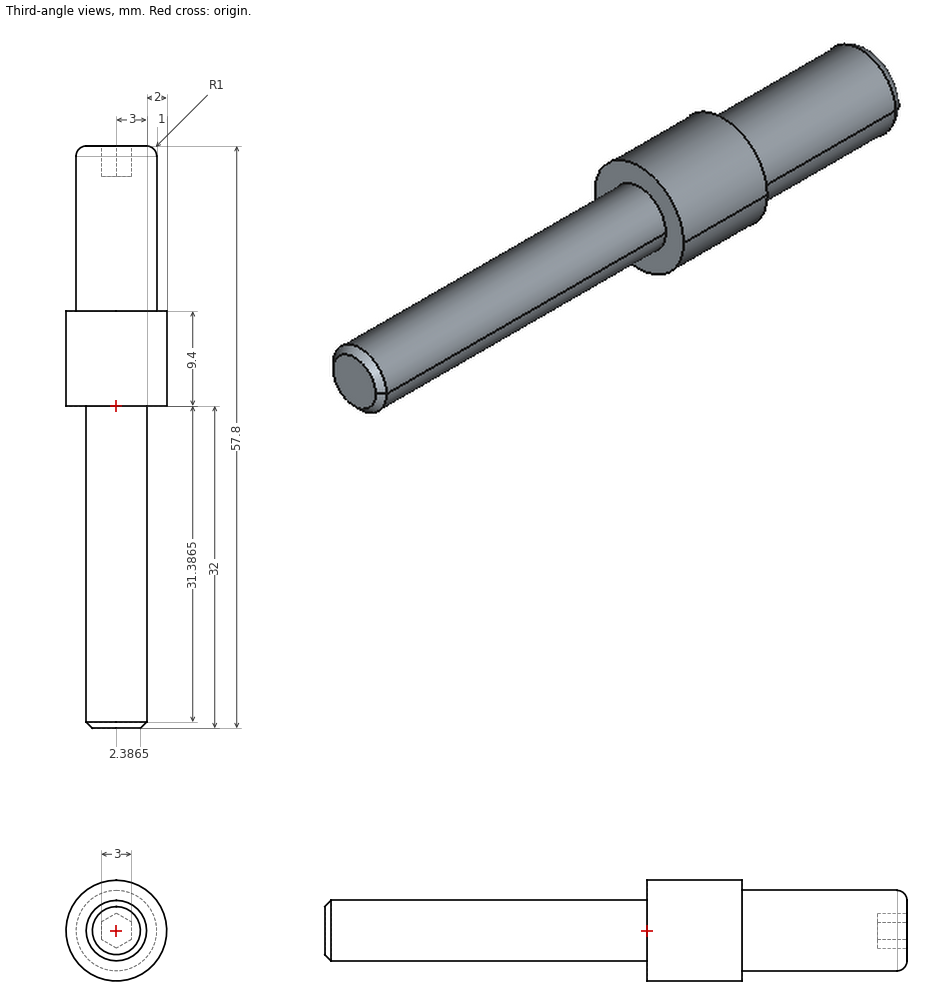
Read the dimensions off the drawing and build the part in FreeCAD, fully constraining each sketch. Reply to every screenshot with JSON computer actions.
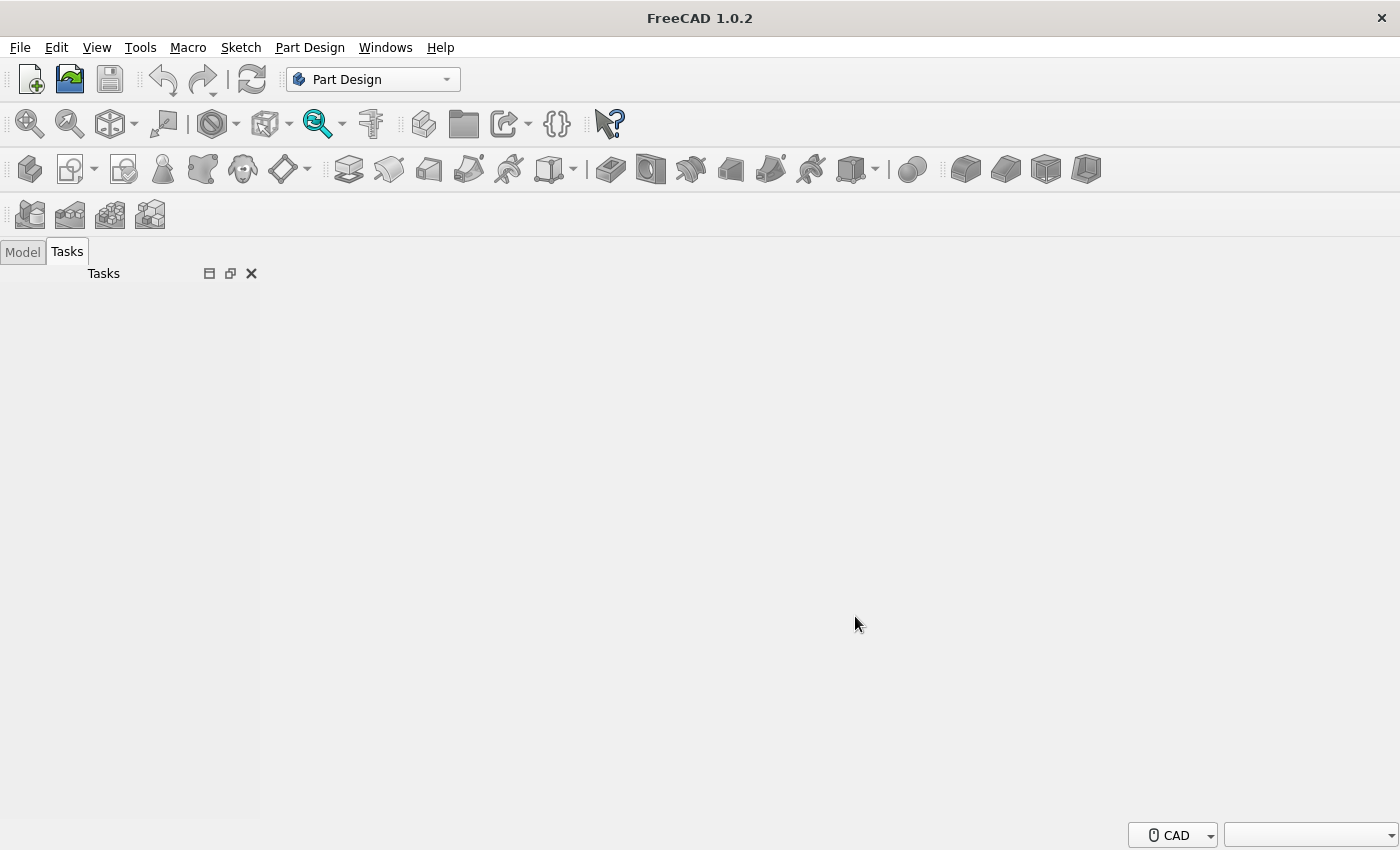
{"action": "left_click", "coordinate": [30, 80]}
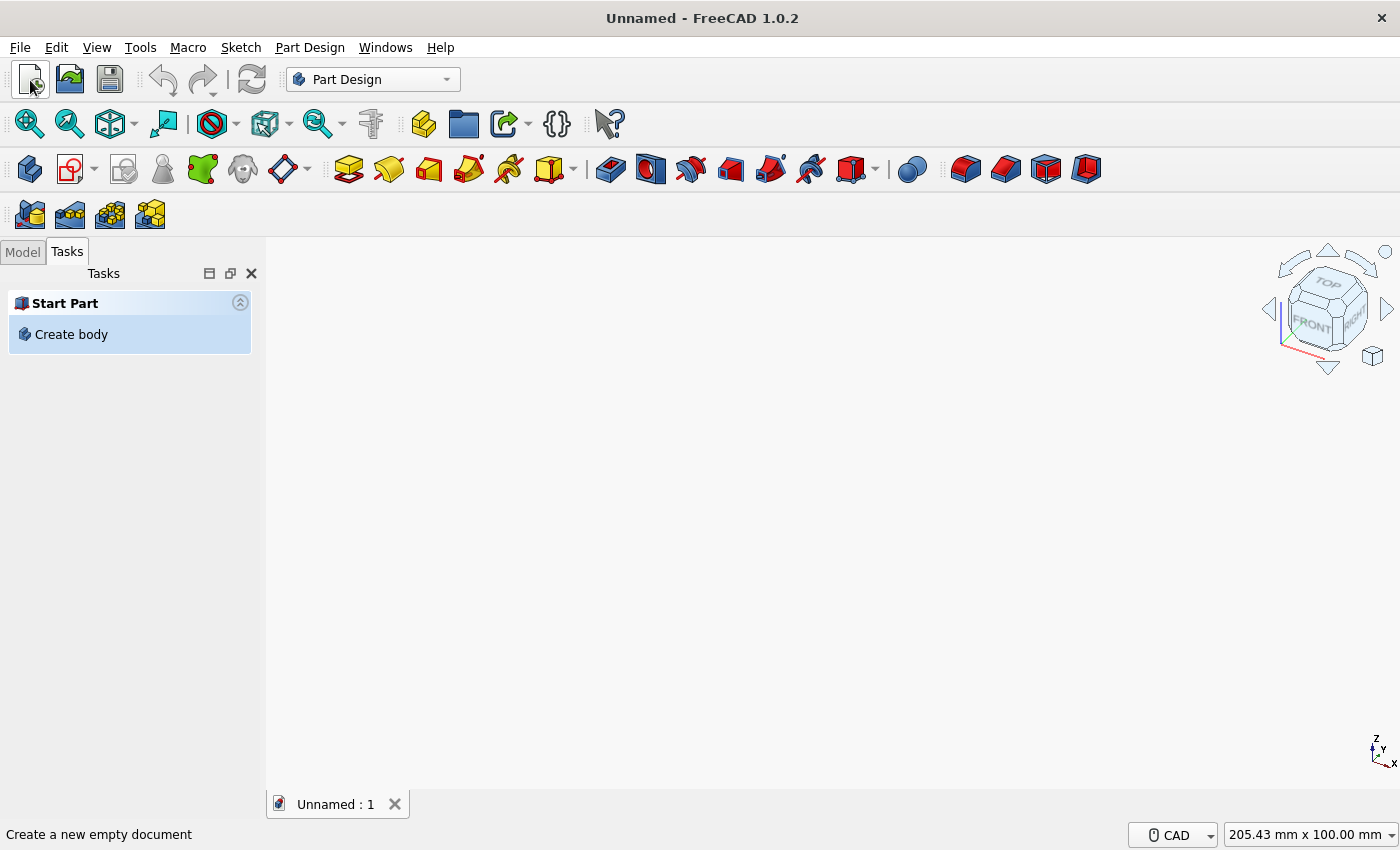
{"action": "left_click", "coordinate": [70, 170]}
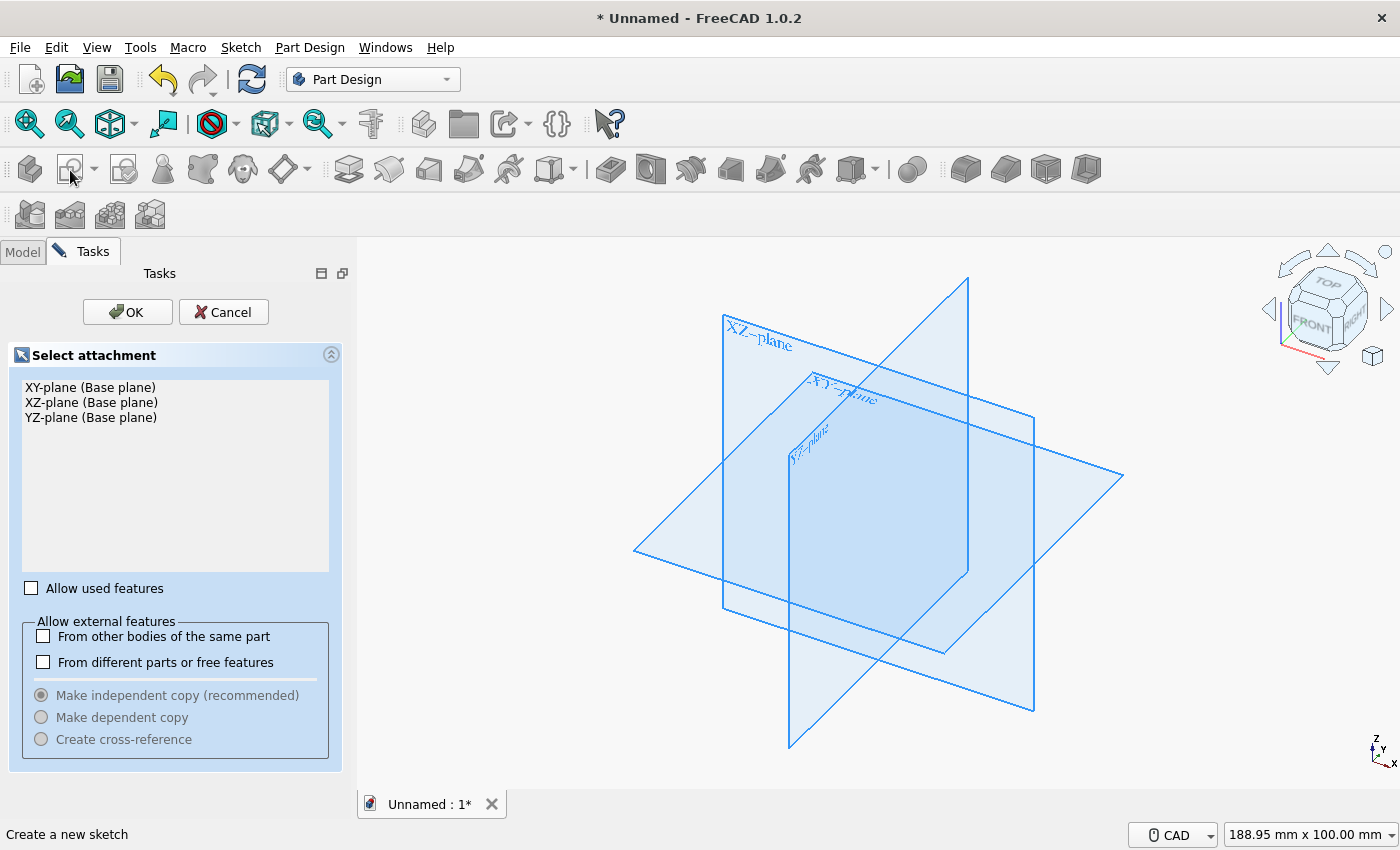
{"action": "left_click", "coordinate": [82, 388]}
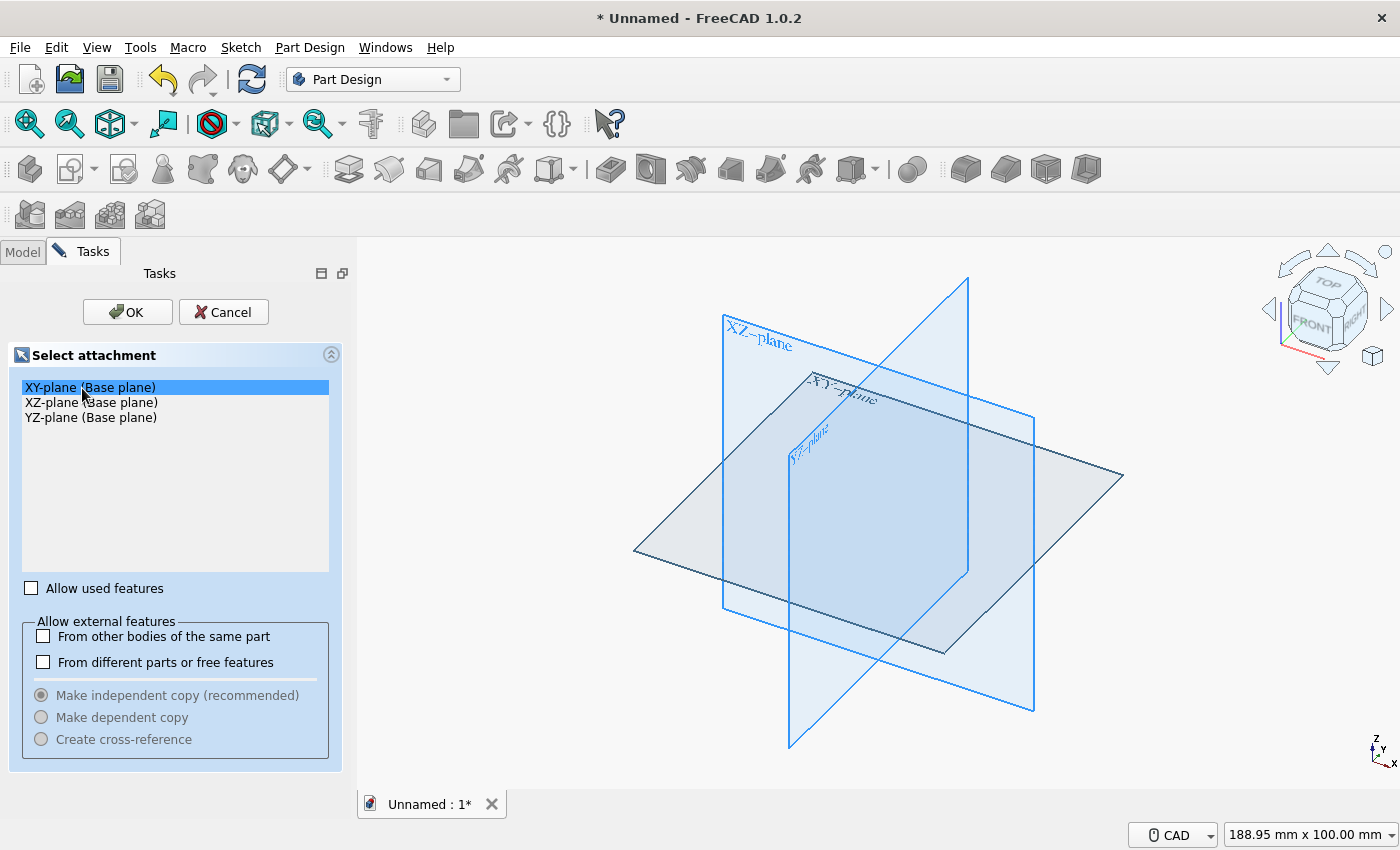
{"action": "left_click", "coordinate": [128, 312]}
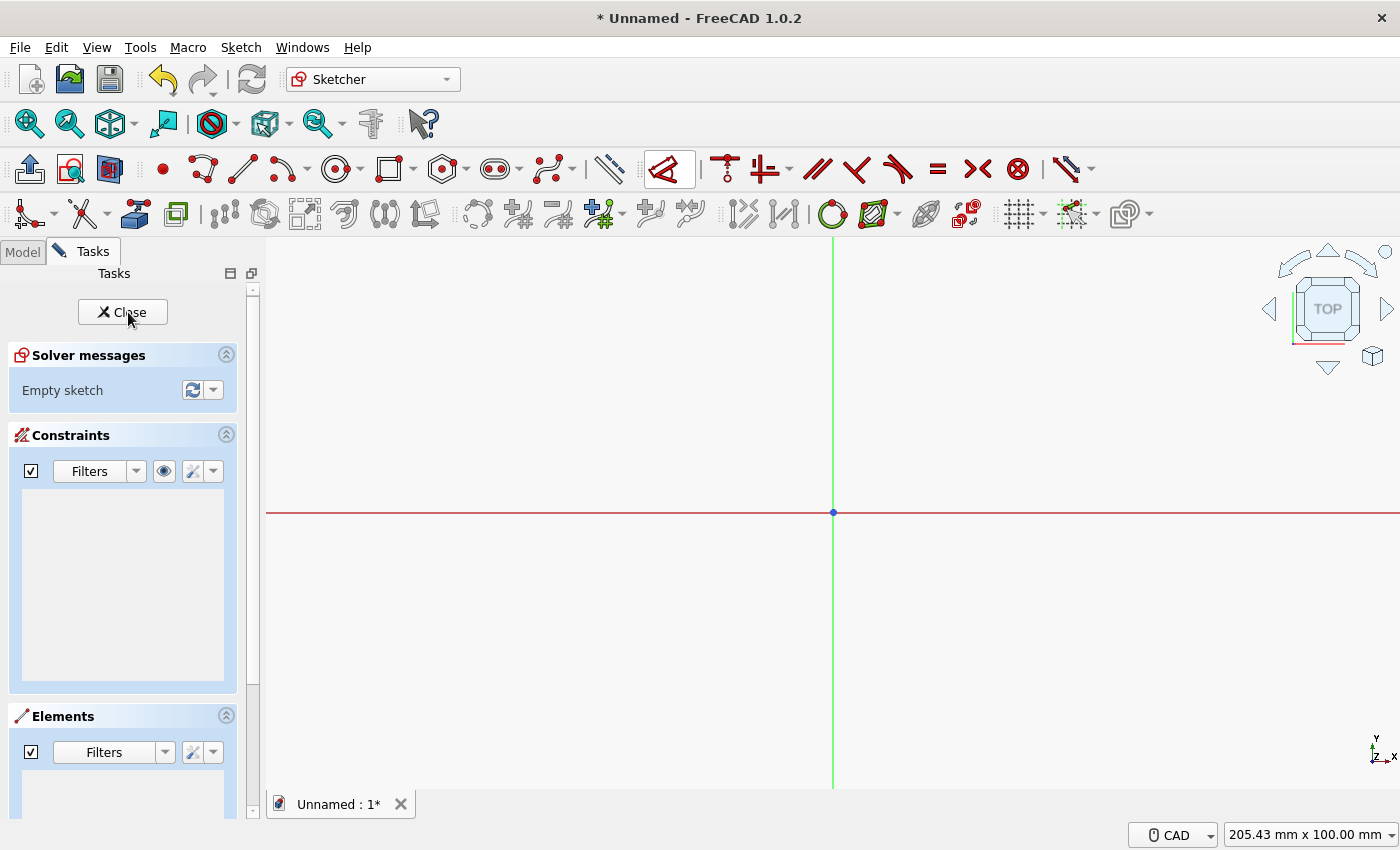
{"action": "left_click", "coordinate": [204, 170]}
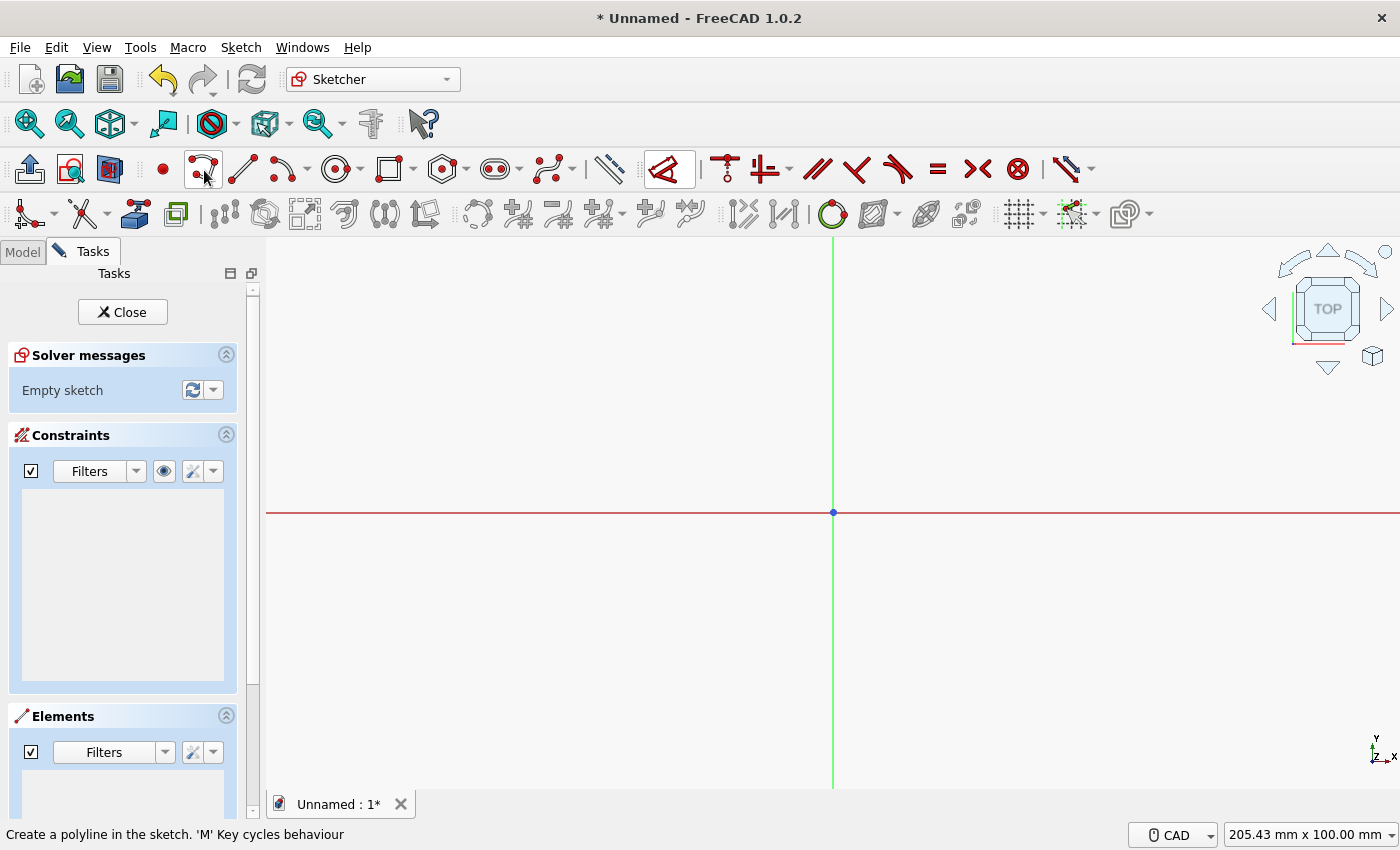
{"action": "left_click", "coordinate": [850, 371]}
{"action": "left_click", "coordinate": [833, 371]}
{"action": "left_click", "coordinate": [842, 690]}
{"action": "left_click", "coordinate": [846, 690]}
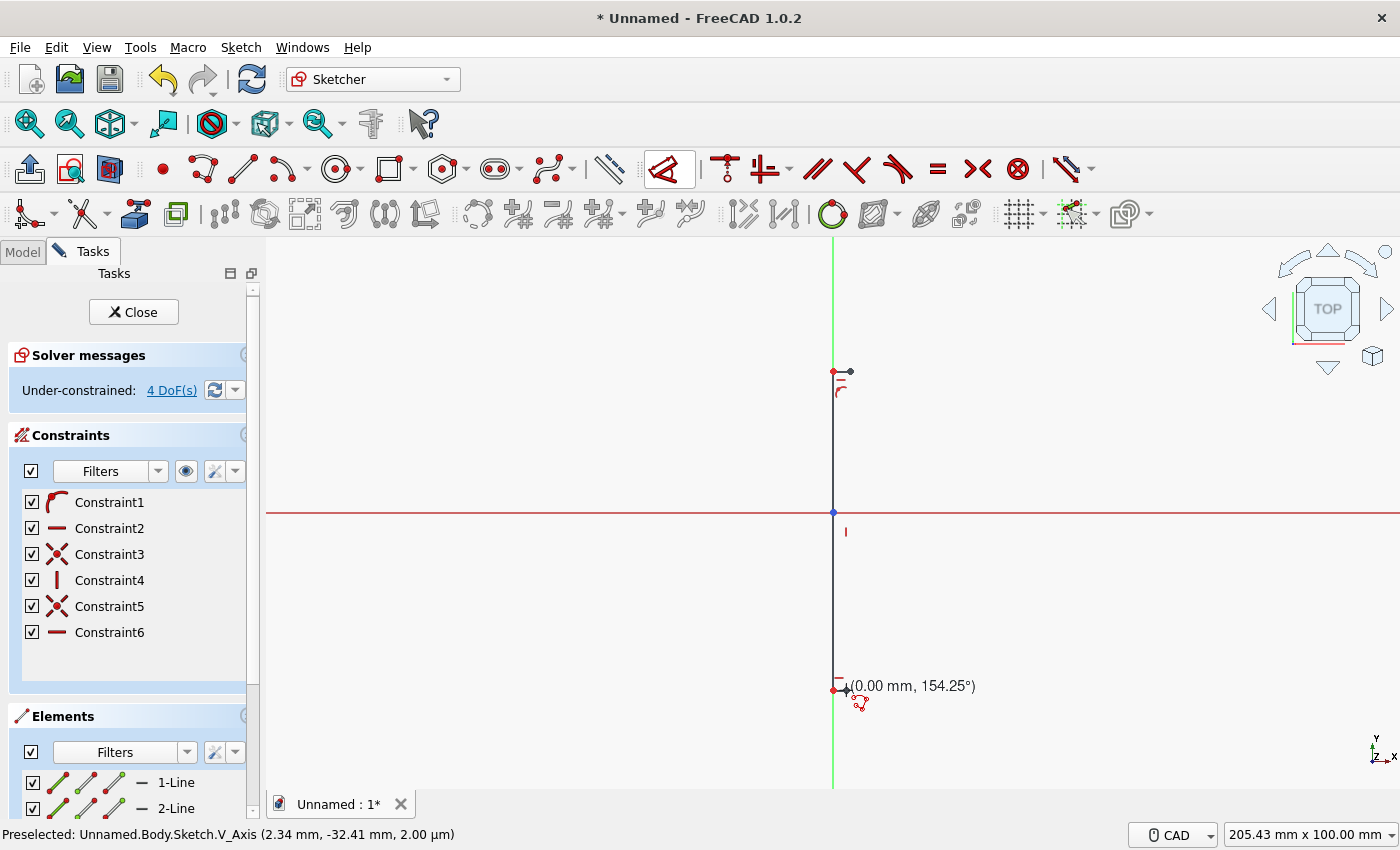
{"action": "scroll", "coordinate": [850, 686], "scroll_direction": "up", "scroll_amount": 6}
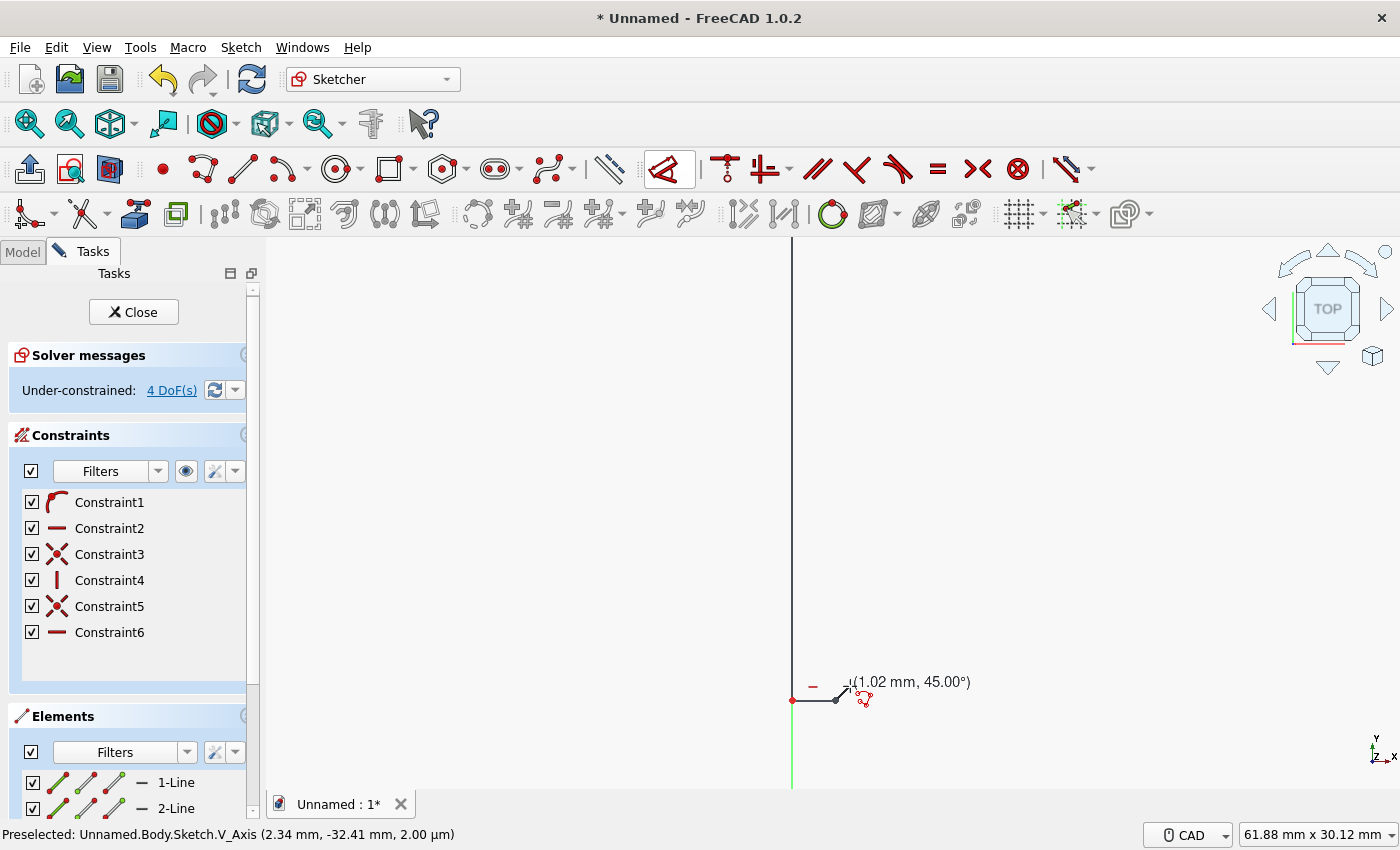
{"action": "left_click", "coordinate": [847, 685]}